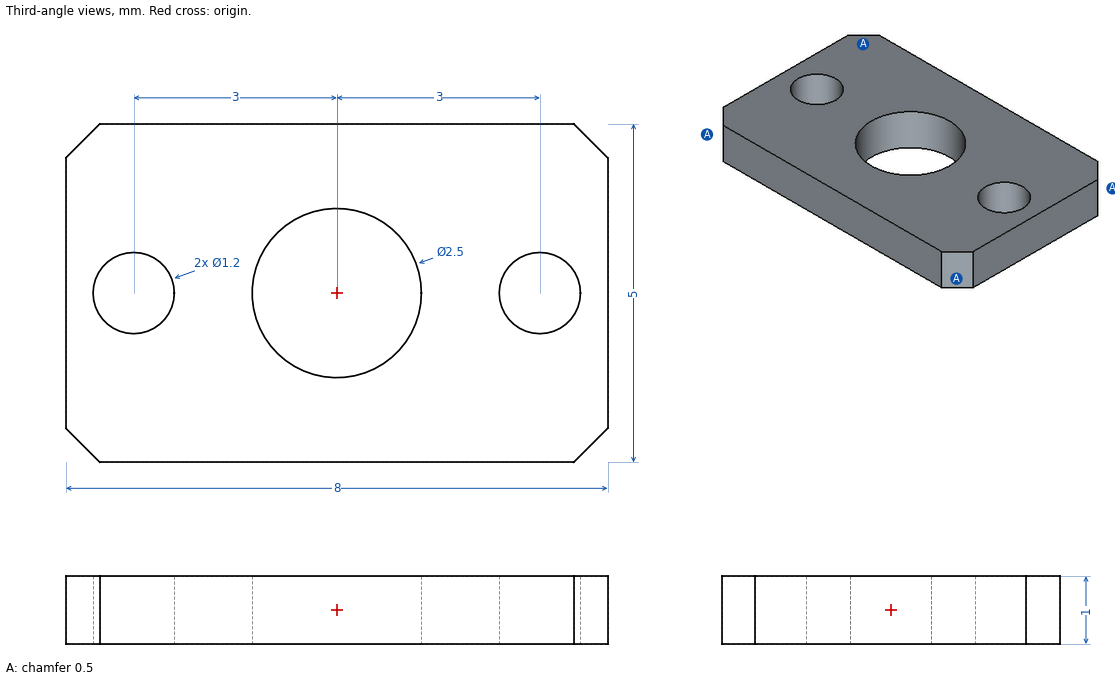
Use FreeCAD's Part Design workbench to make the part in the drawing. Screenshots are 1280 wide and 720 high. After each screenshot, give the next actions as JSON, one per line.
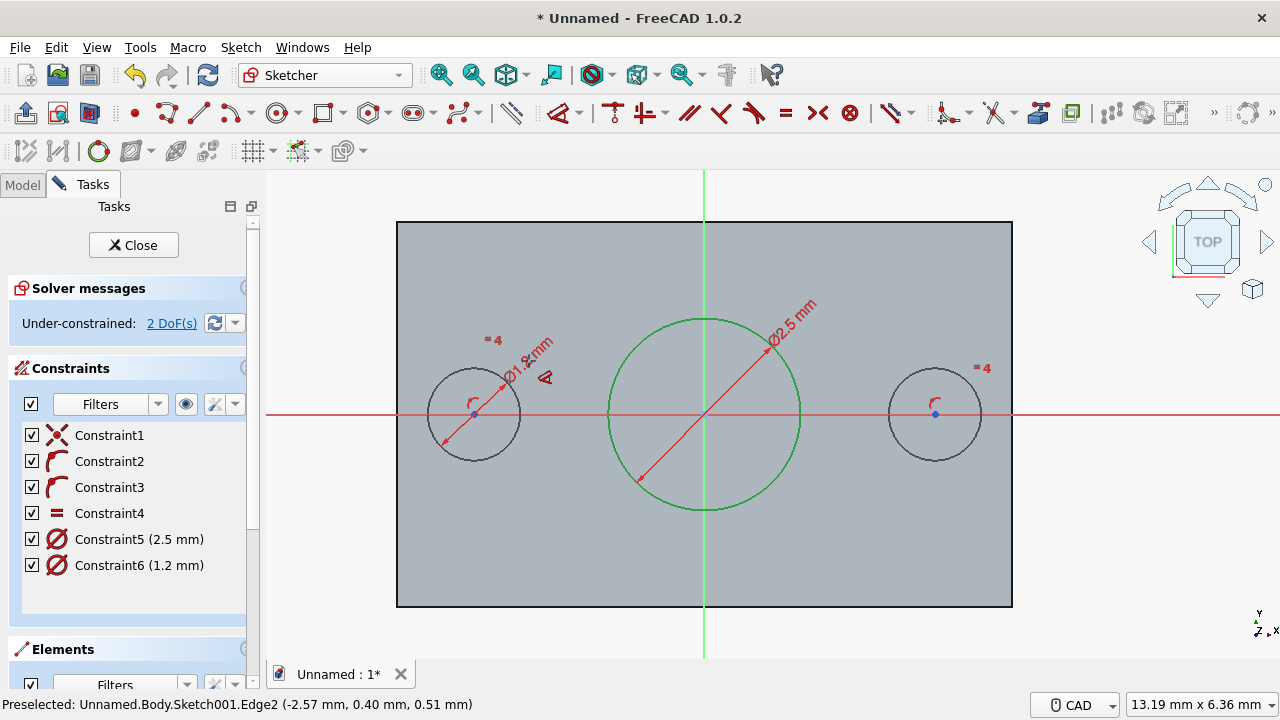
{"action": "left_click", "coordinate": [474, 414]}
{"action": "left_click", "coordinate": [589, 448]}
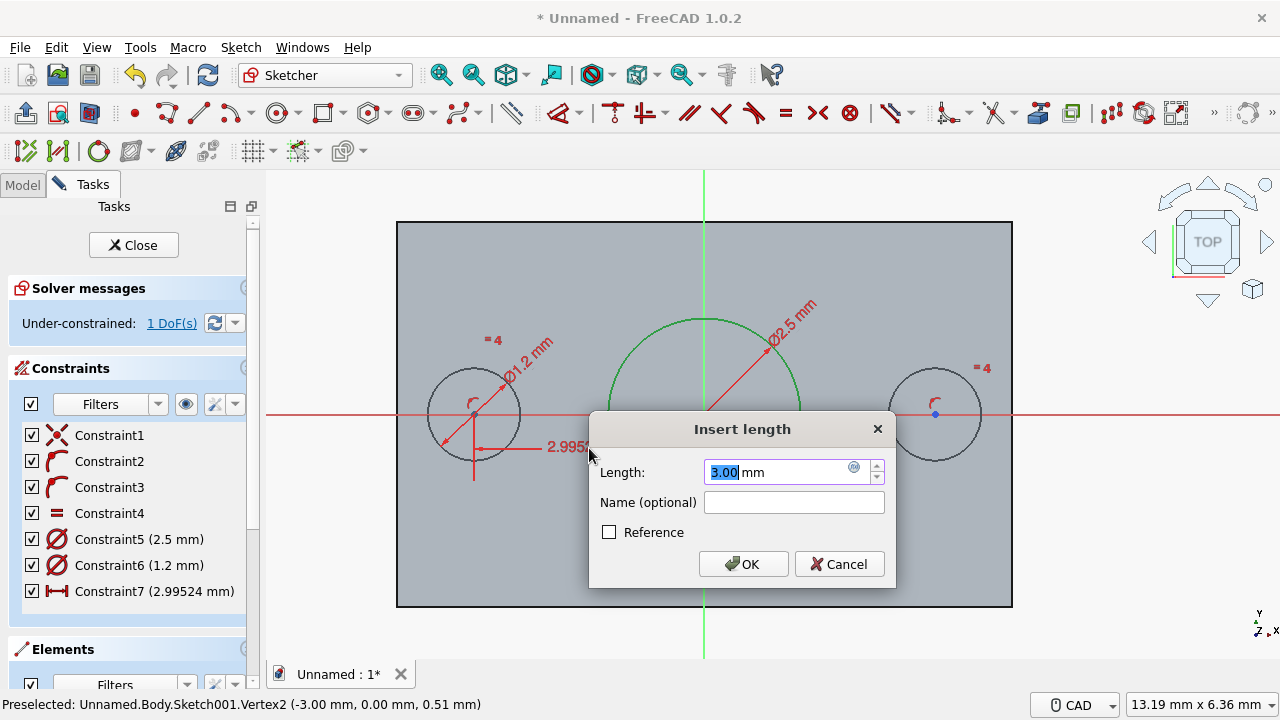
{"action": "type", "text": "3"}
{"action": "key", "text": "Return"}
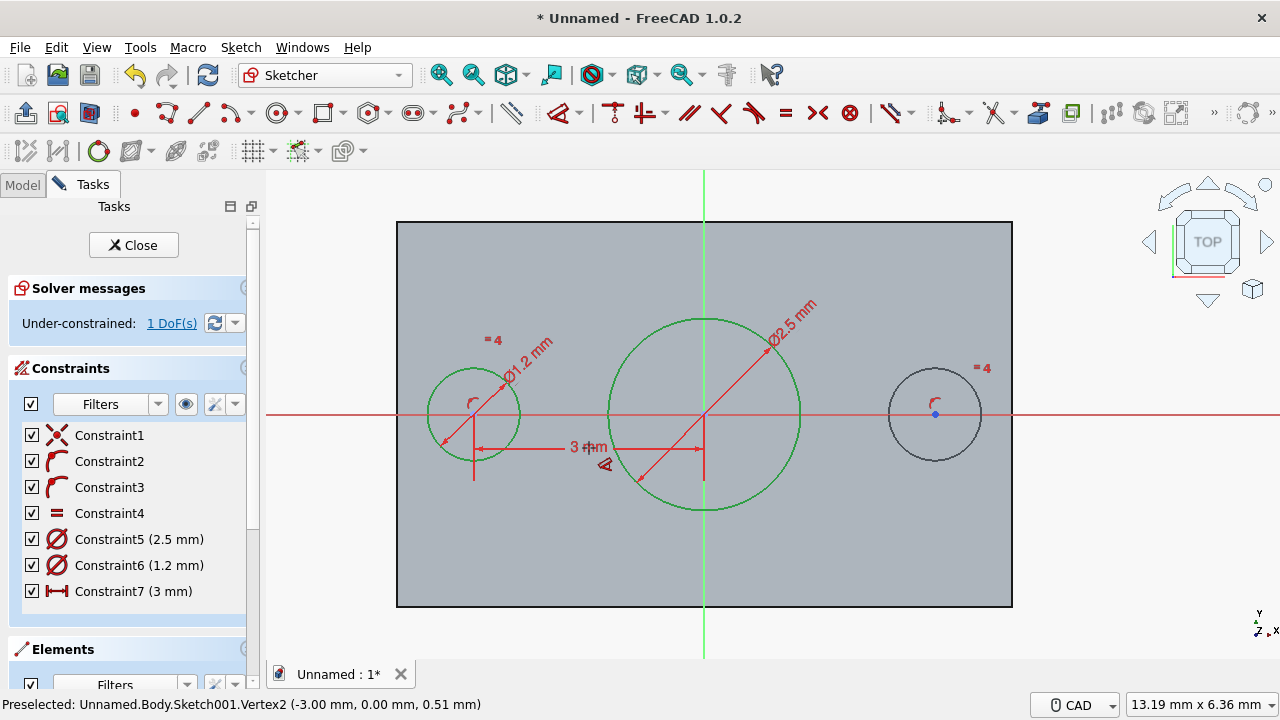
{"action": "left_click", "coordinate": [935, 414]}
{"action": "left_click", "coordinate": [820, 448]}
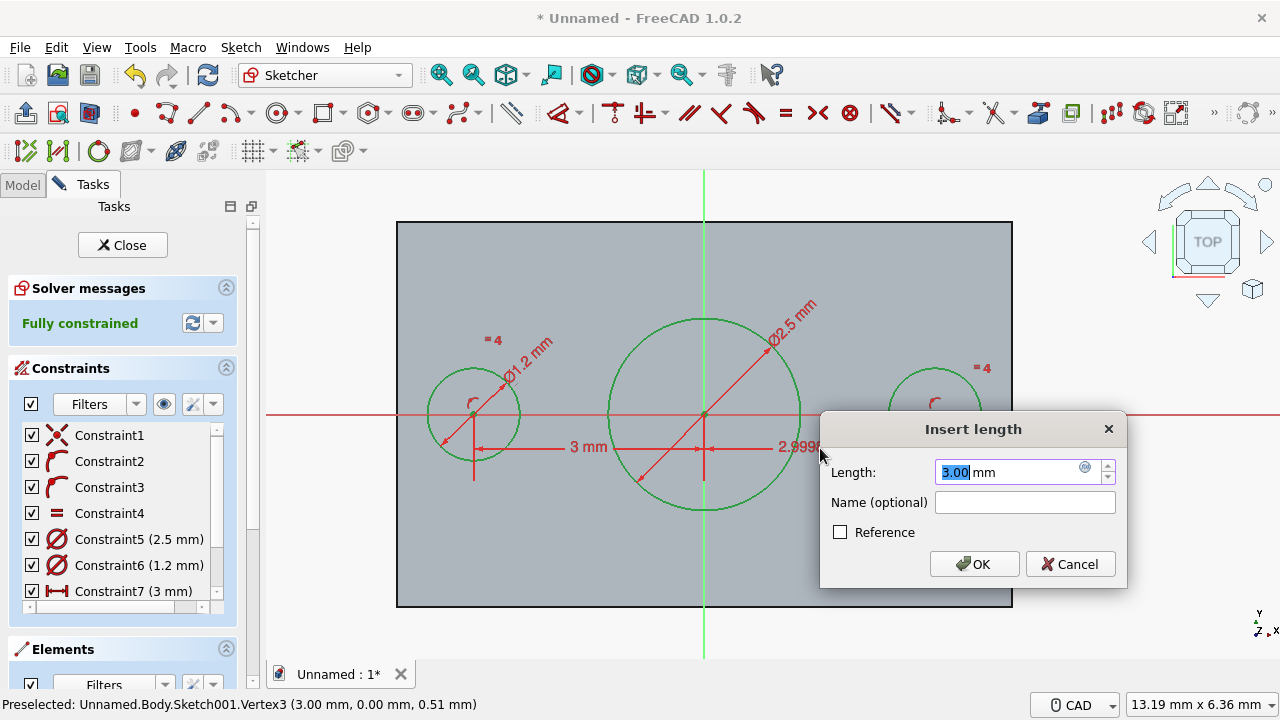
{"action": "type", "text": "3"}
{"action": "key", "text": "Return"}
{"action": "key", "text": "Escape"}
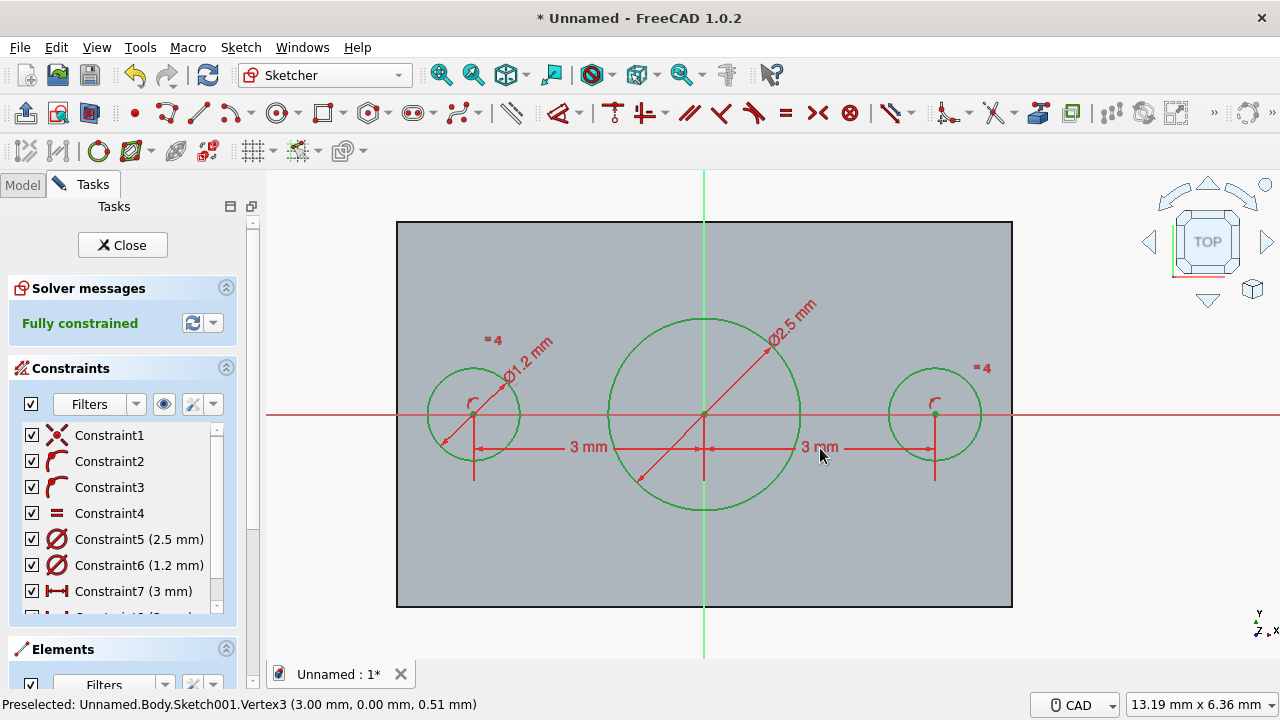
{"action": "left_click", "coordinate": [123, 245]}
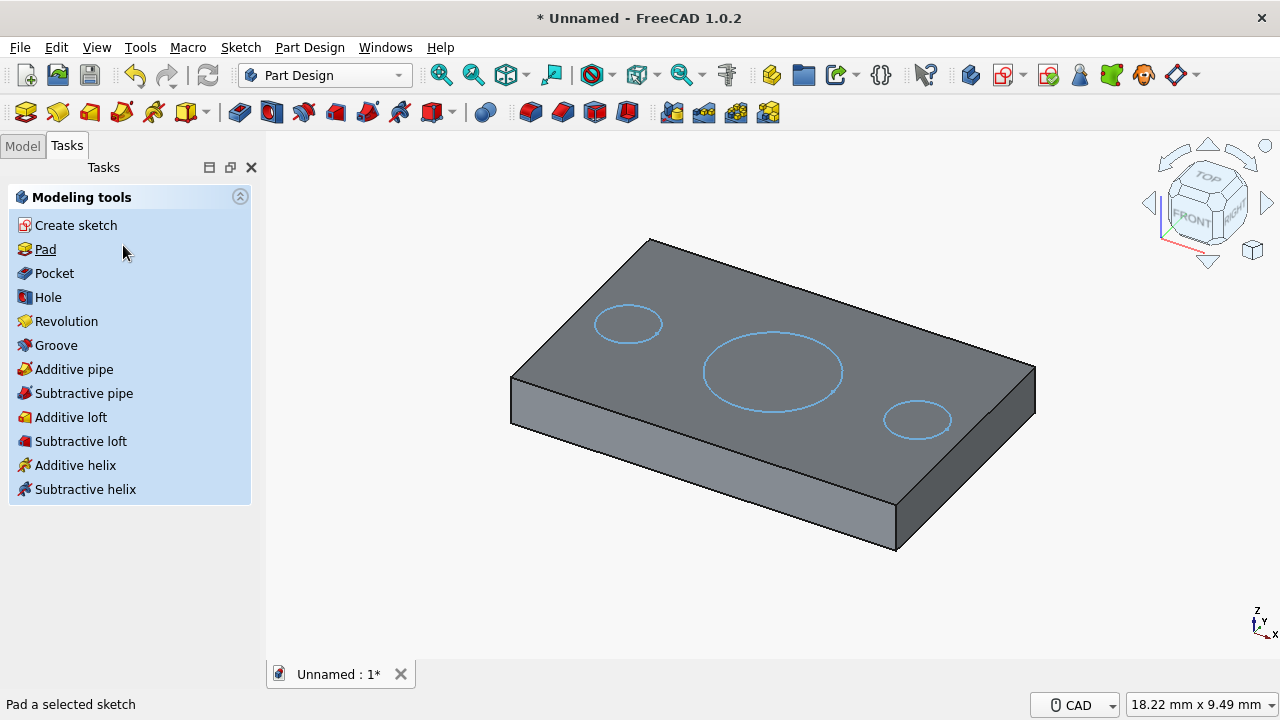
{"action": "left_click", "coordinate": [240, 112]}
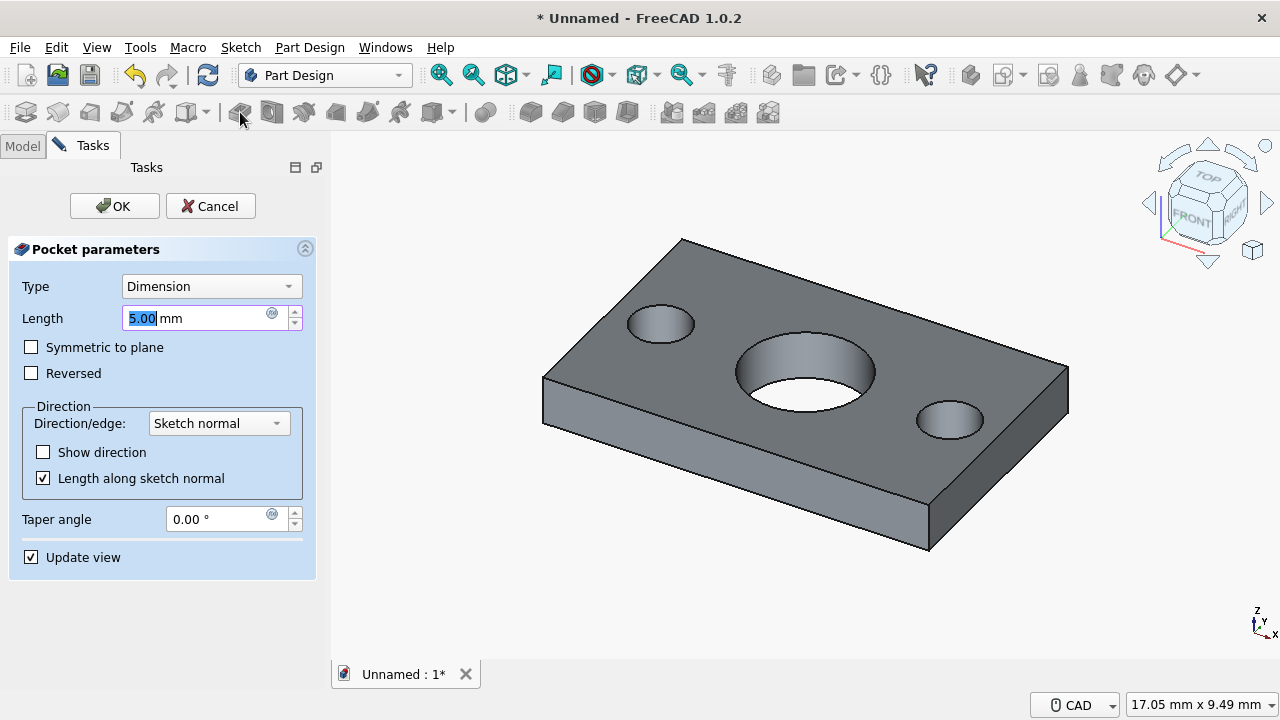
{"action": "left_click", "coordinate": [212, 286]}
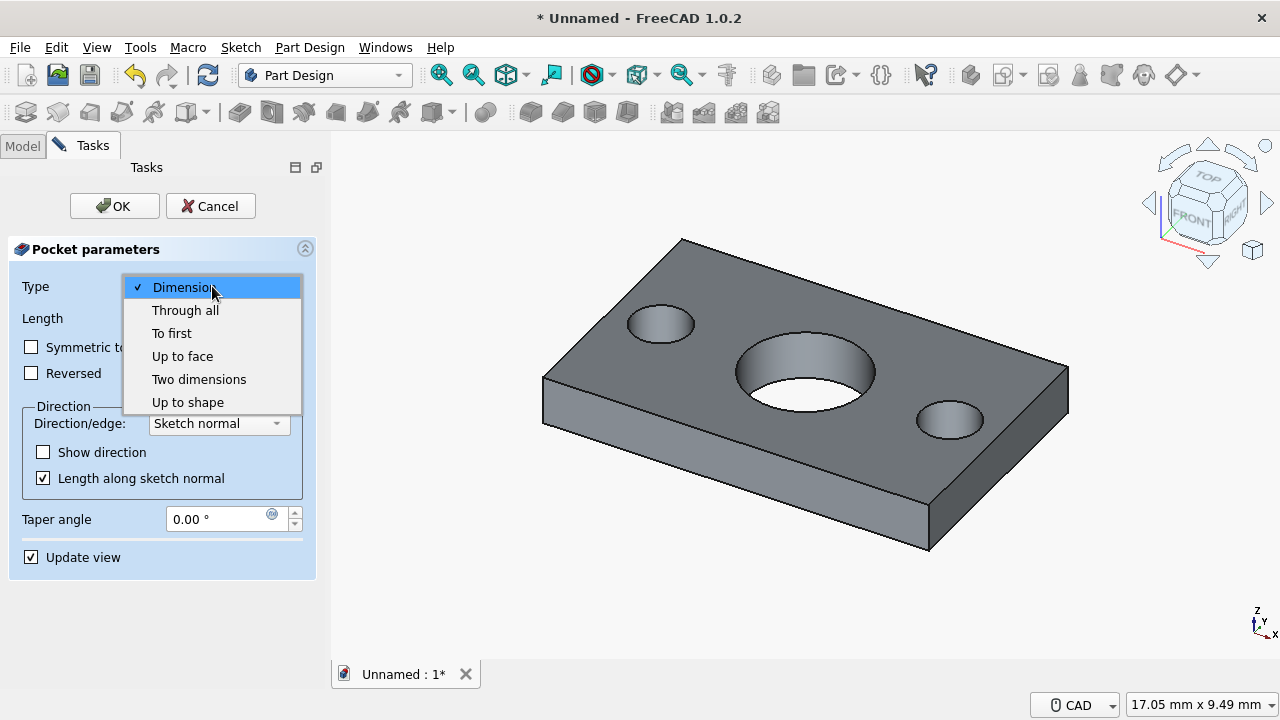
{"action": "left_click", "coordinate": [212, 310]}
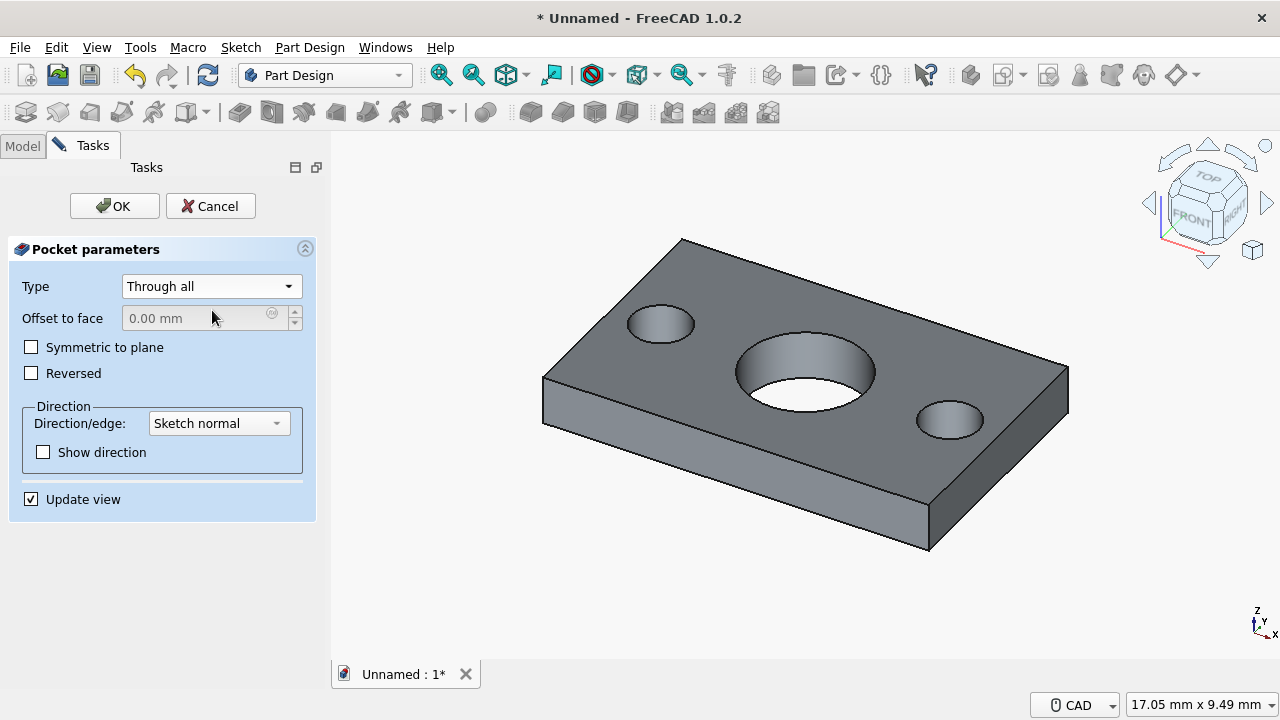
{"action": "left_click", "coordinate": [115, 206]}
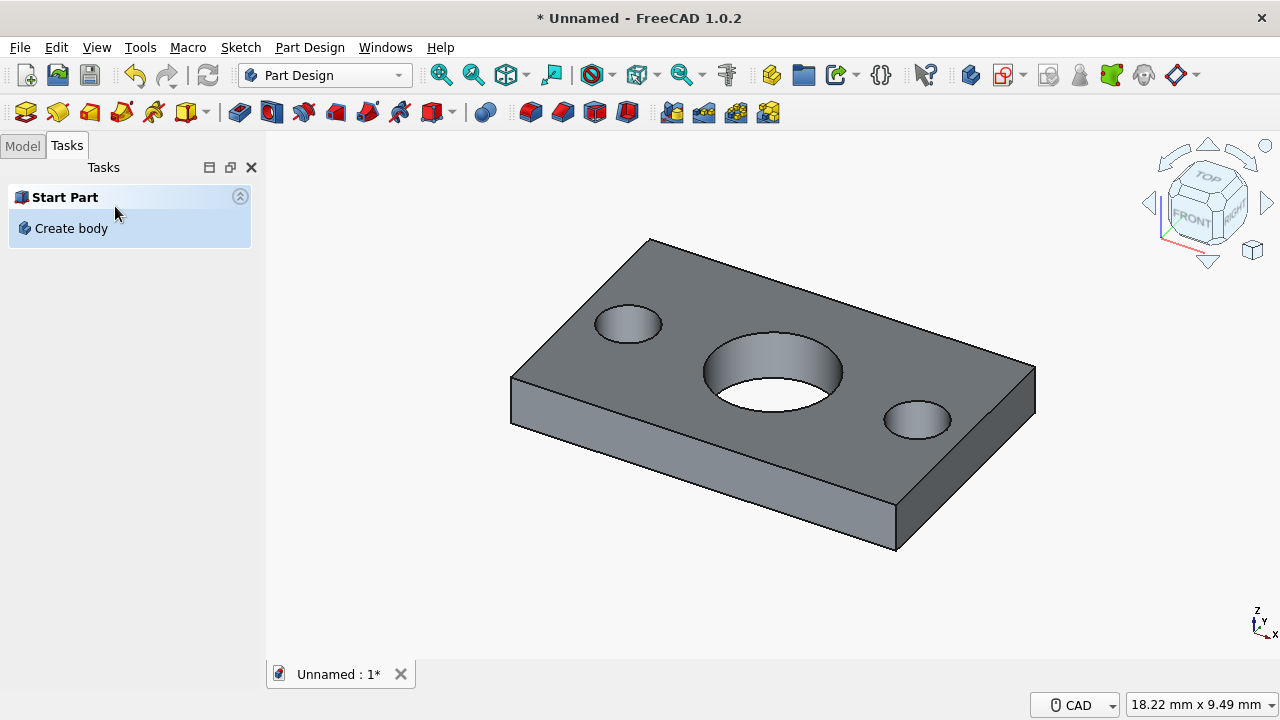
{"action": "left_click", "coordinate": [896, 527]}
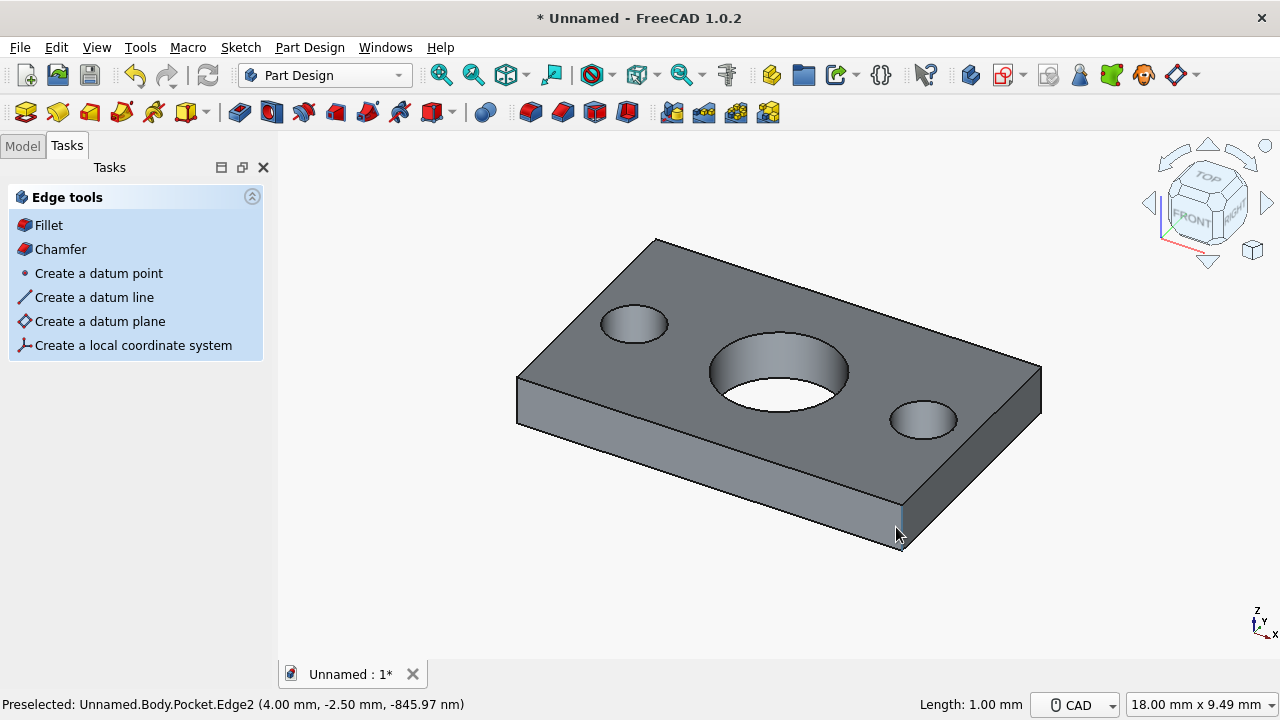
{"action": "key", "text": "0"}